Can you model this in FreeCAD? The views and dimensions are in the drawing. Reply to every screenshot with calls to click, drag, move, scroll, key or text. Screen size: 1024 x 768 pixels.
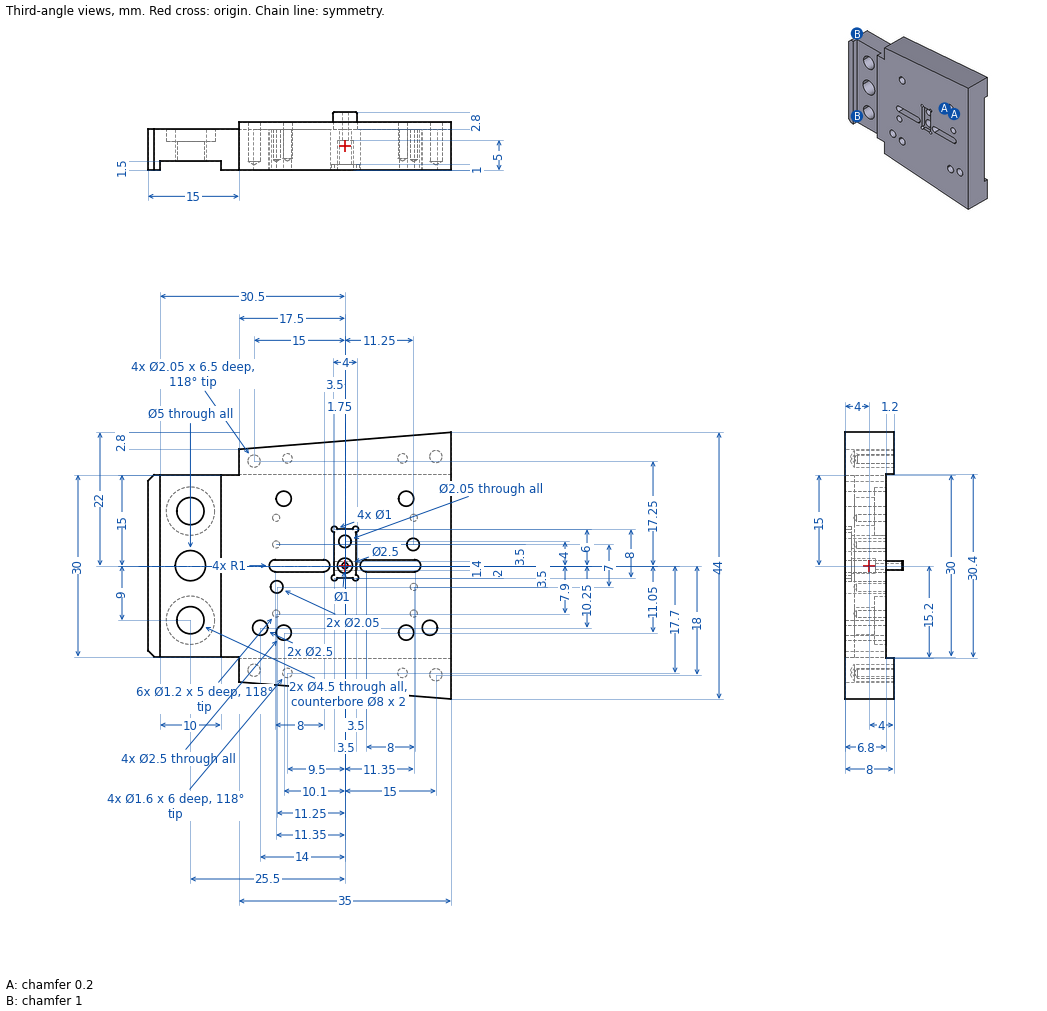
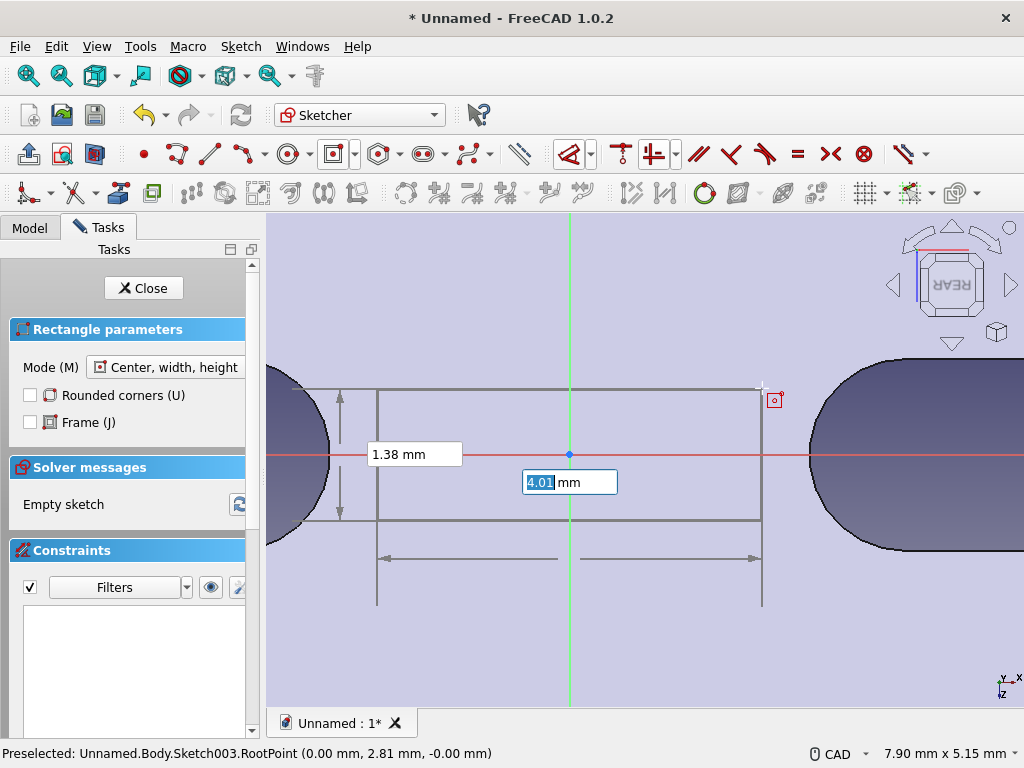
text(4)
key(Tab)
text(1.4)
key(Return)
key(Escape)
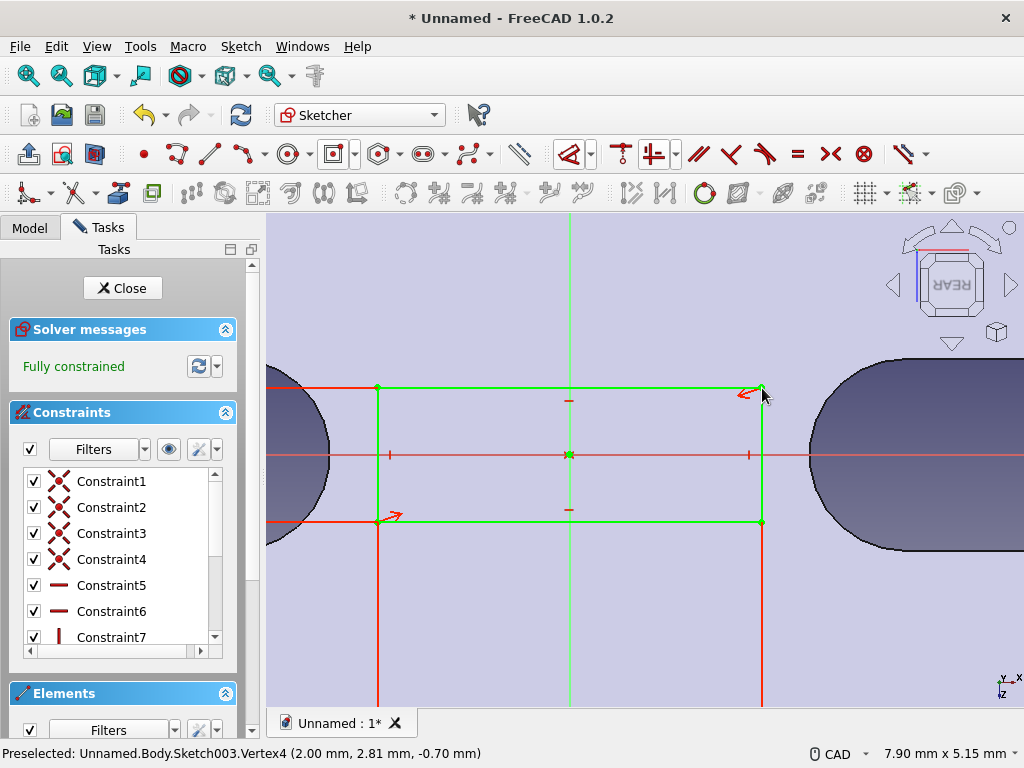
click(123, 288)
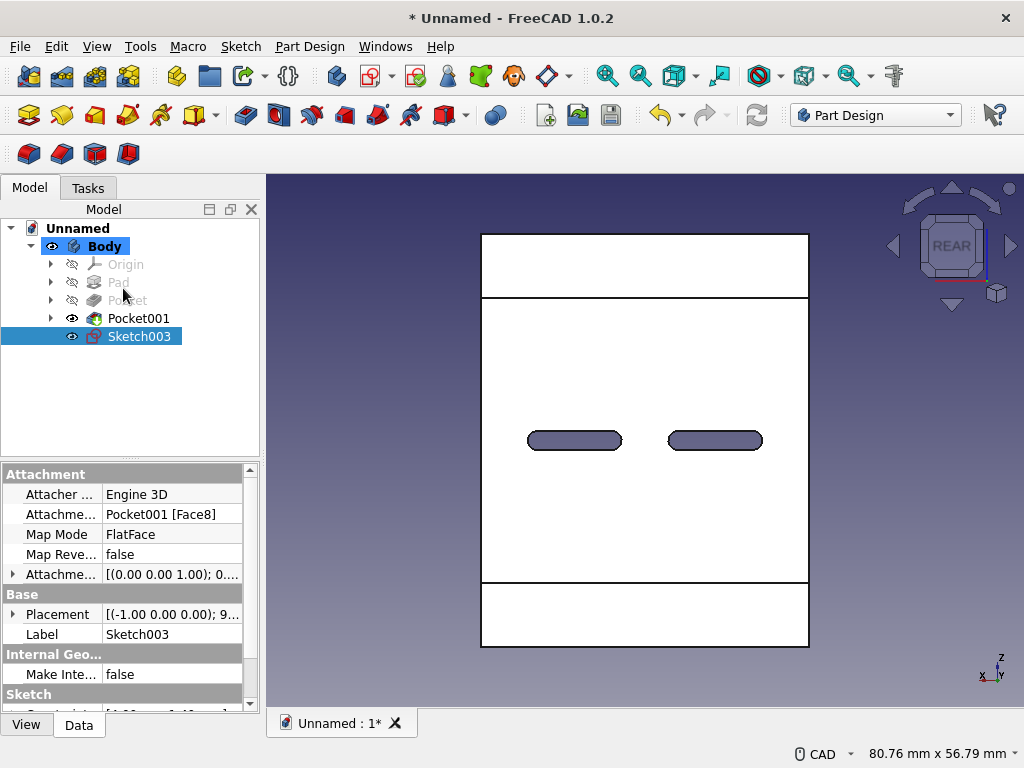
click(29, 116)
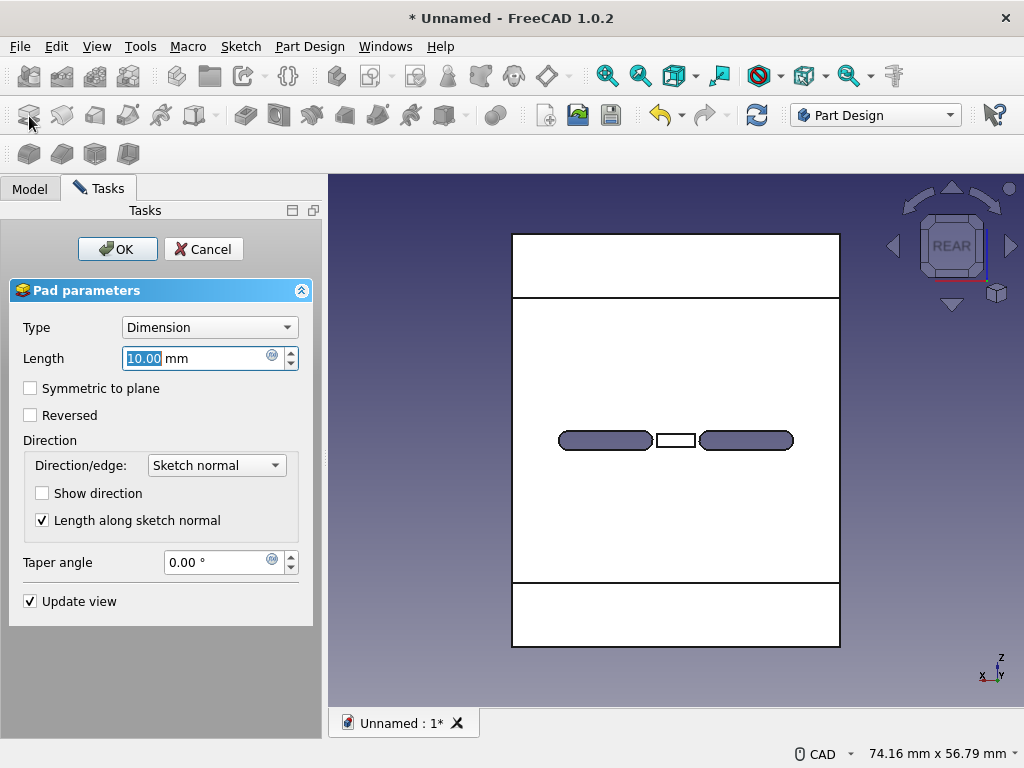
text(2.8)
key(Tab)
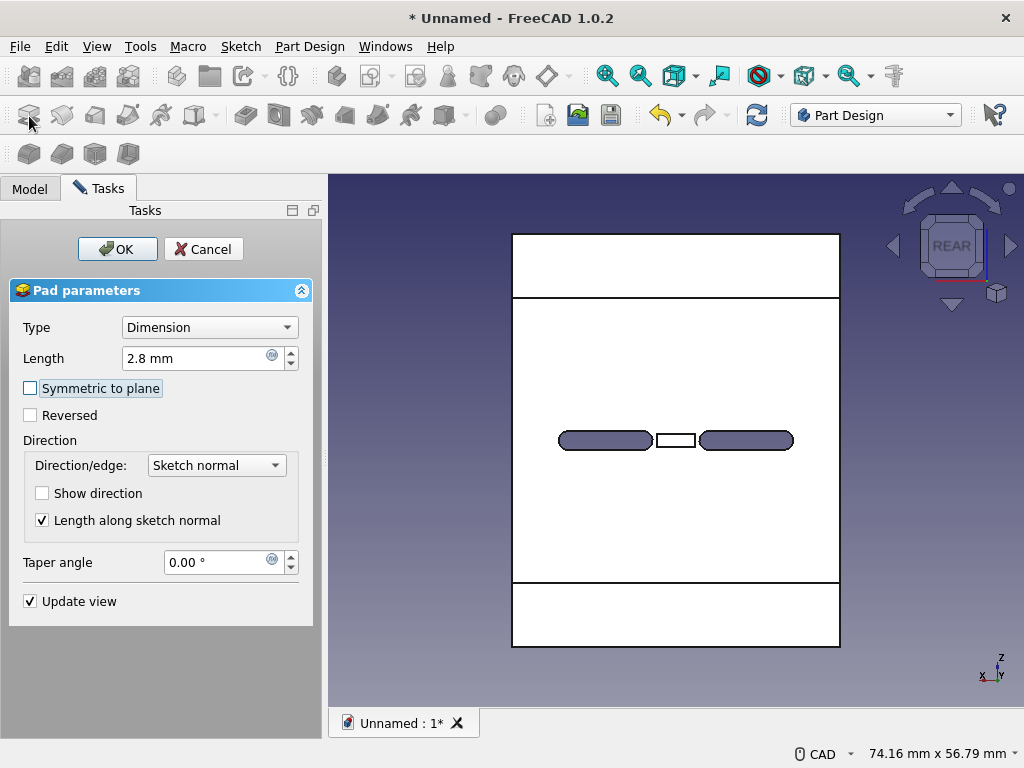
click(118, 249)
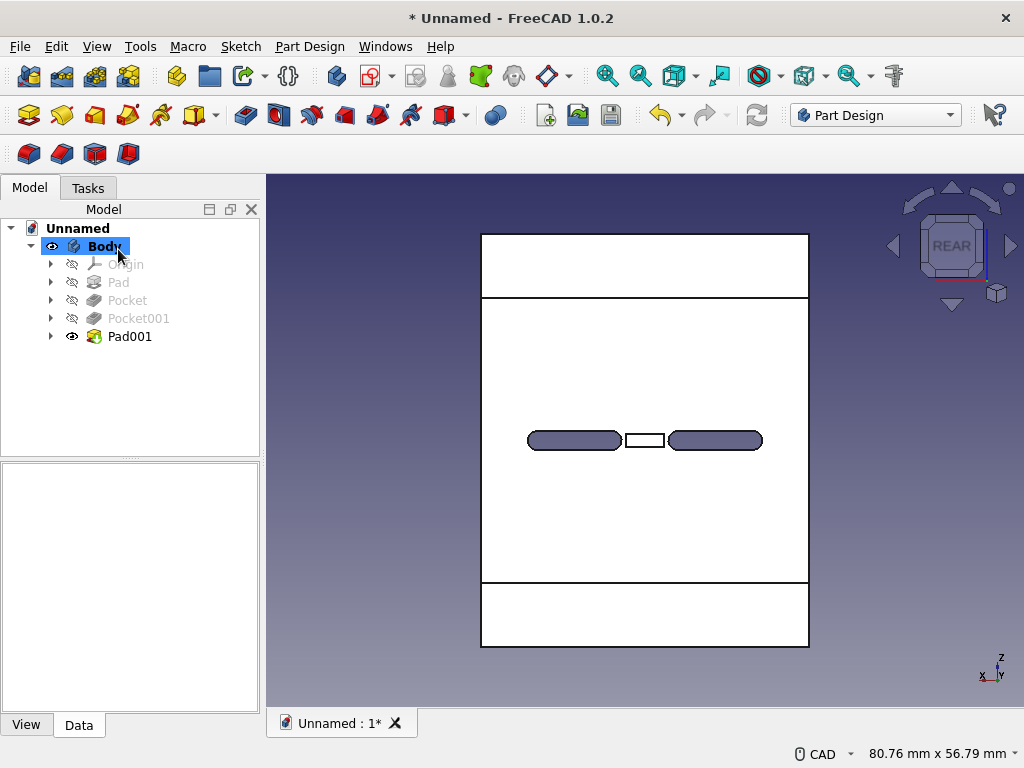
click(664, 440)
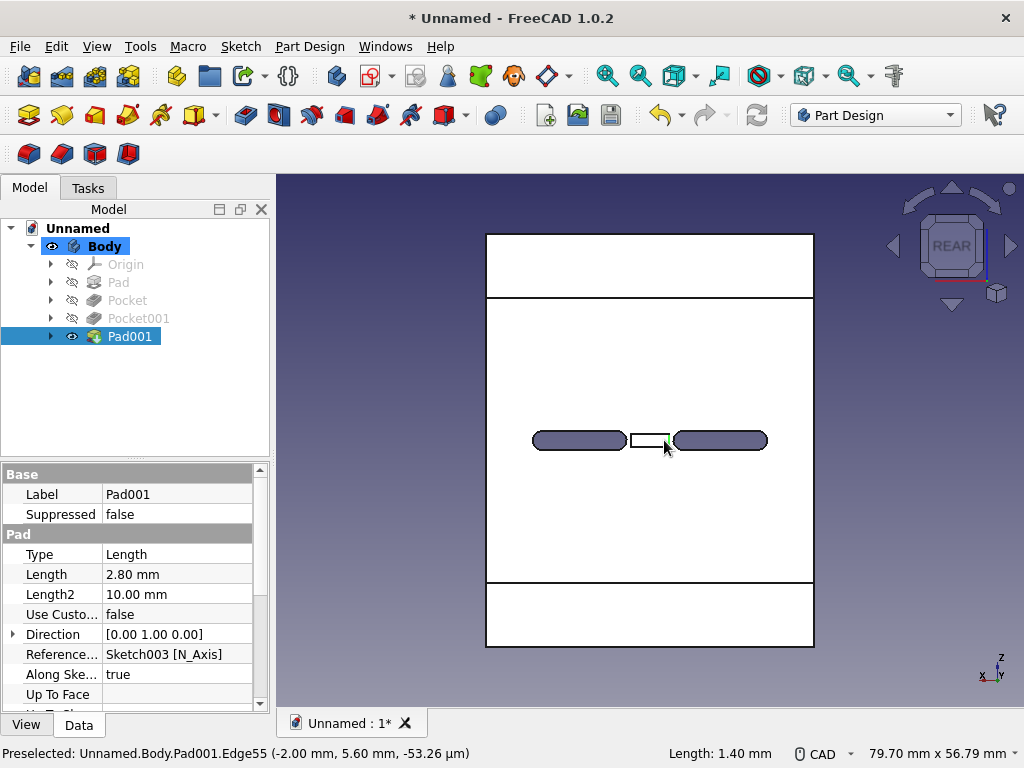
scroll(631, 440, up, 6)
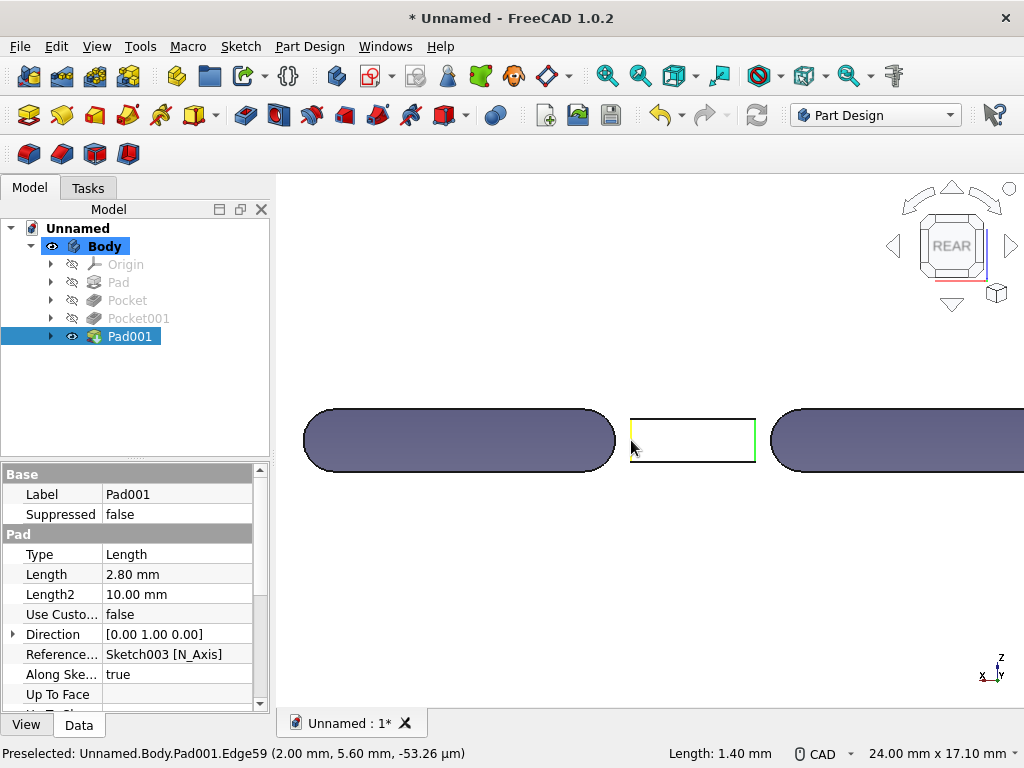
click(608, 76)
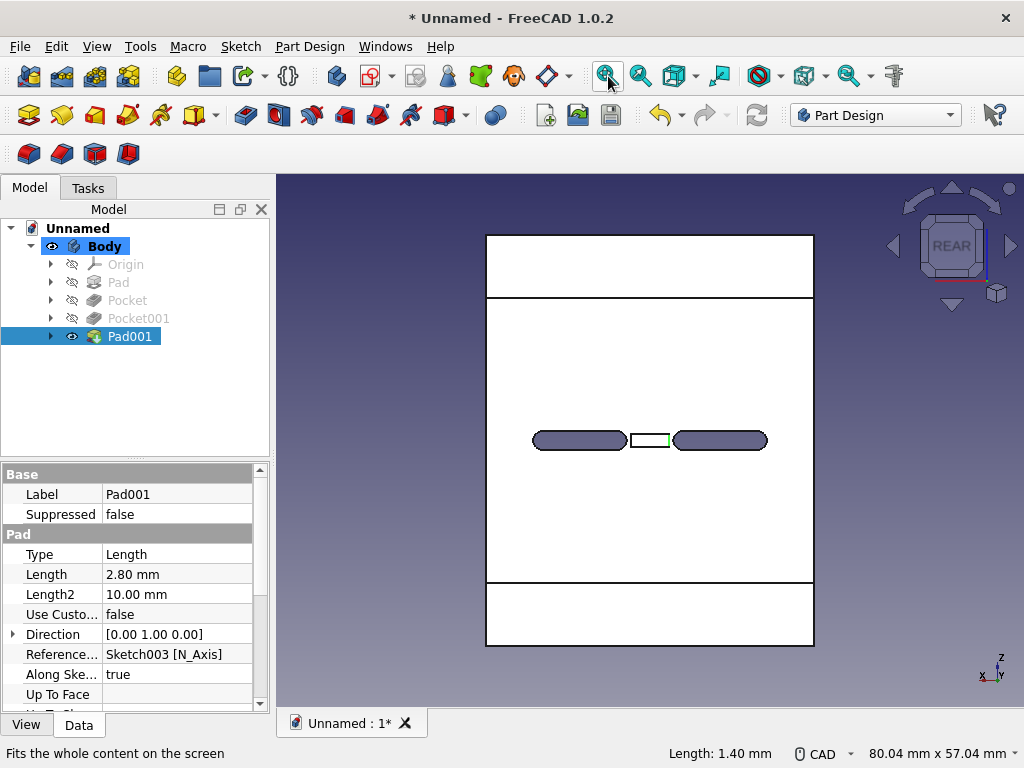
key(0)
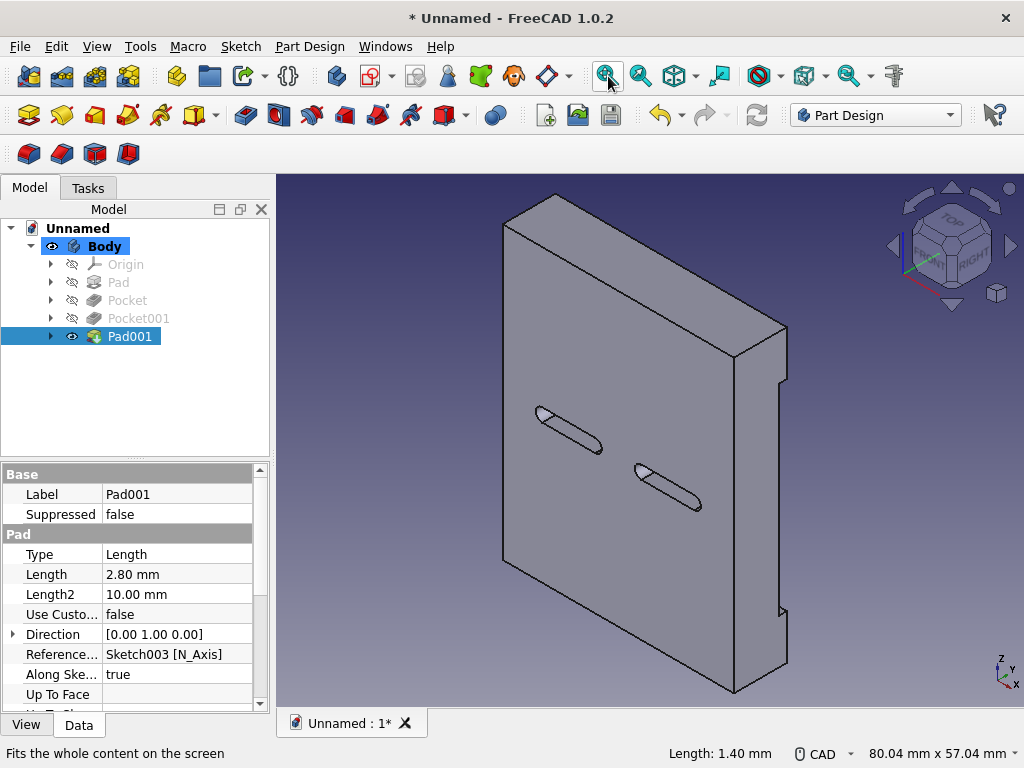
scroll(695, 429, up, 6)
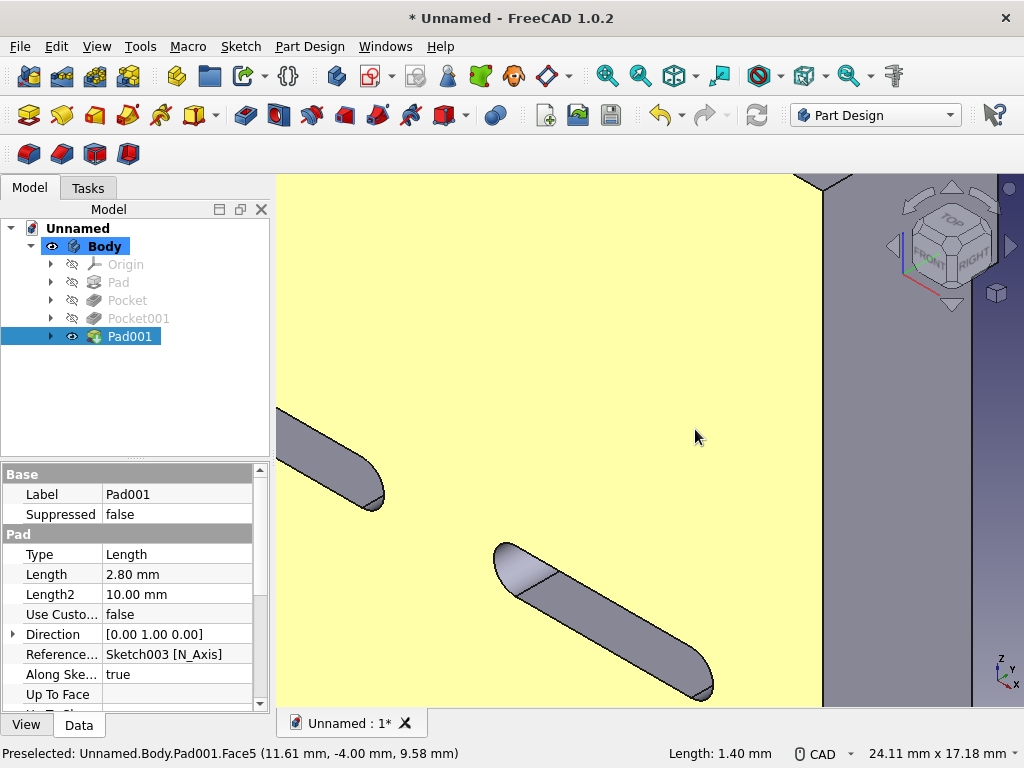
click(608, 76)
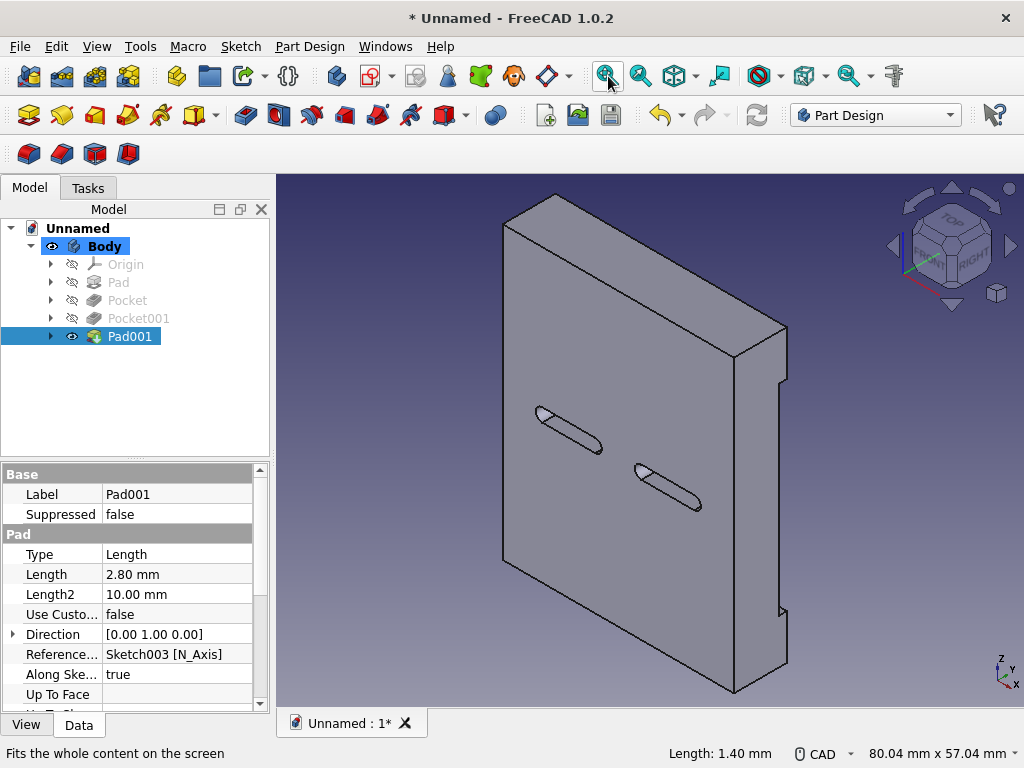
key(2)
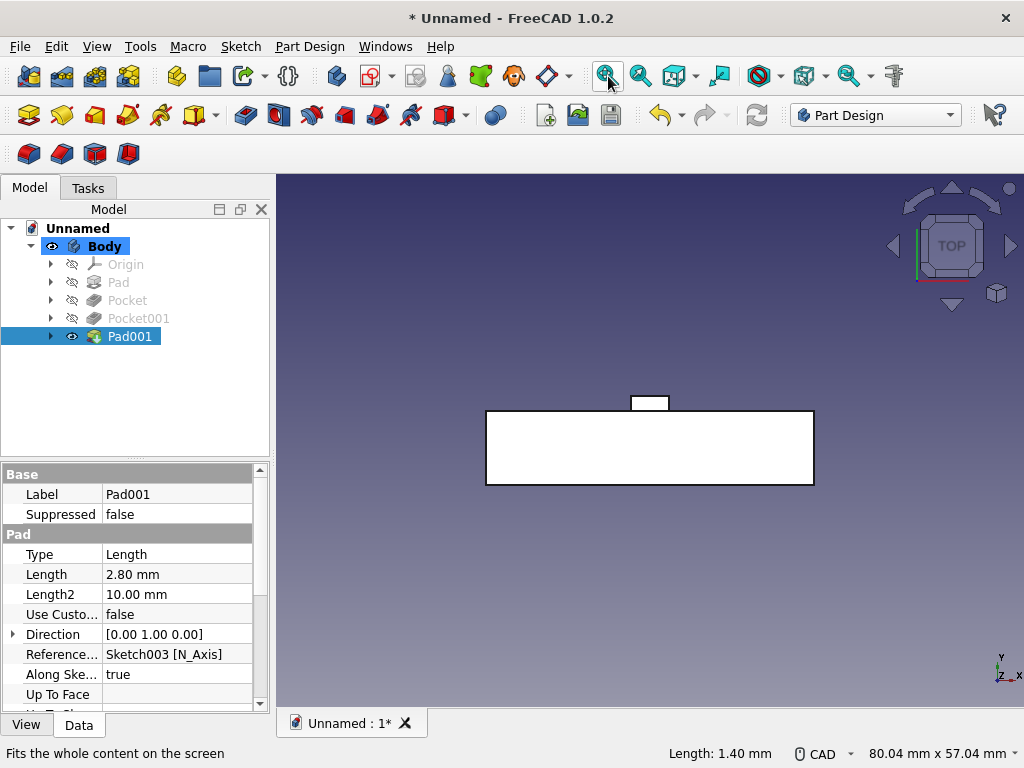
click(608, 76)